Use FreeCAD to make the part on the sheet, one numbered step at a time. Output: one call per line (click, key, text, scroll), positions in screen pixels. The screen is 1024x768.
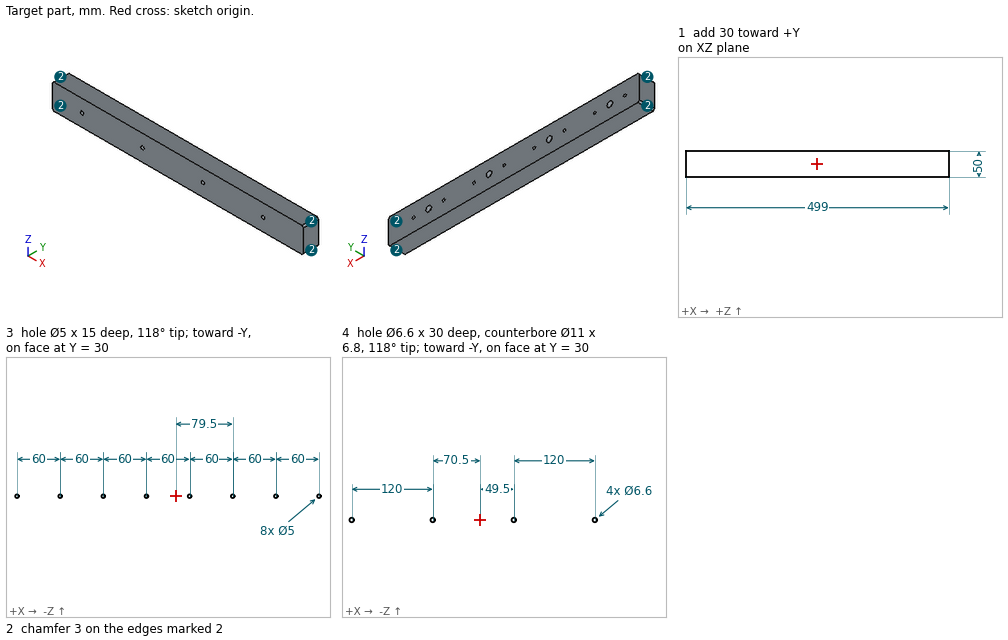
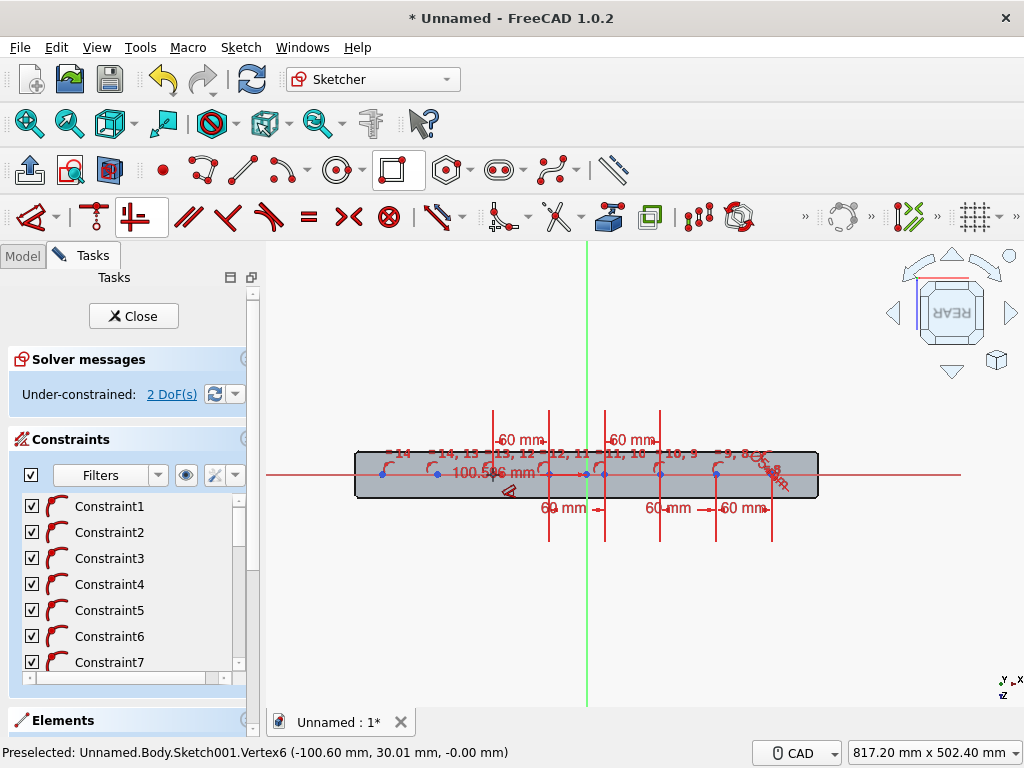
click(438, 475)
click(466, 509)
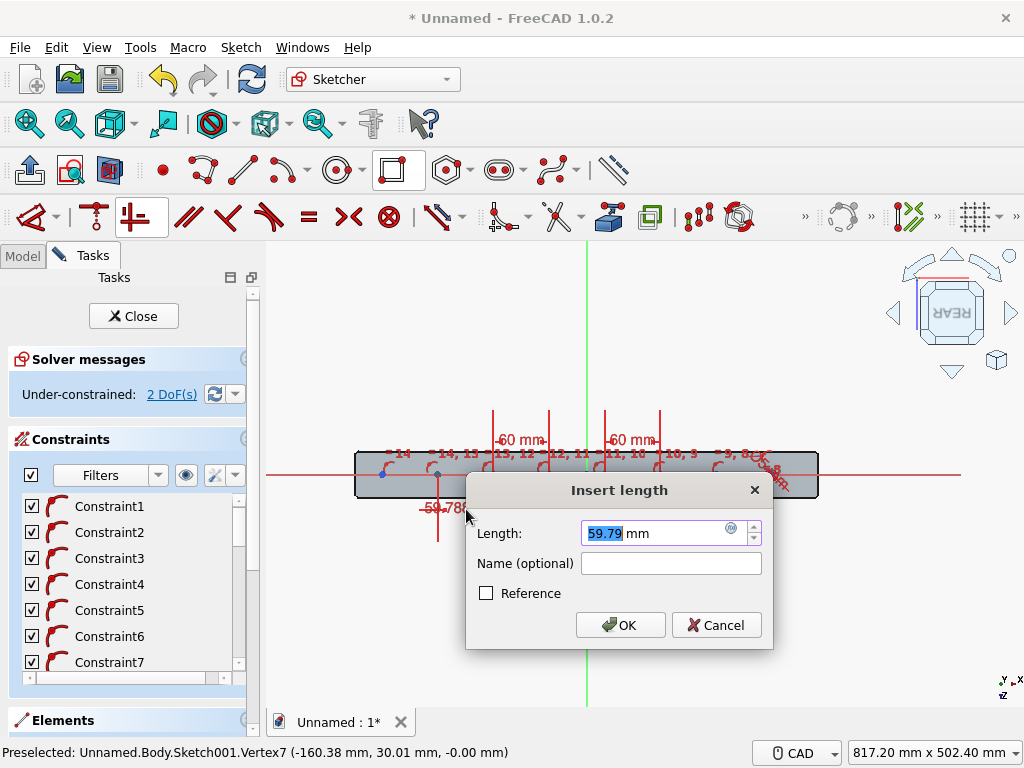
text(60)
key(Return)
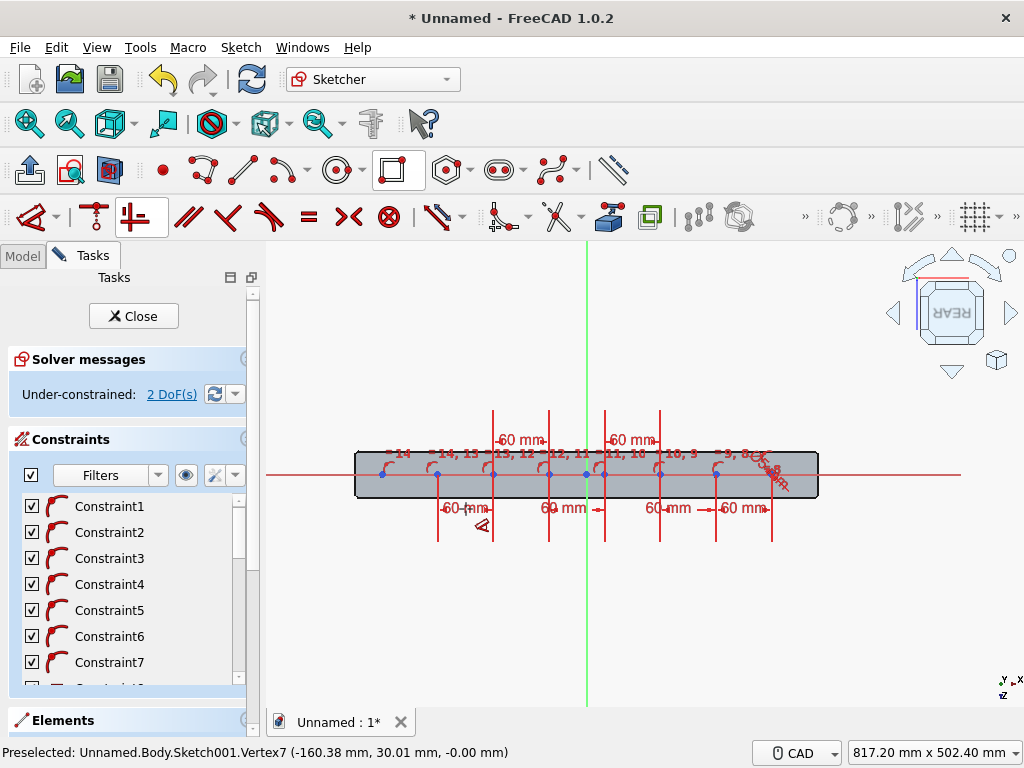
click(438, 475)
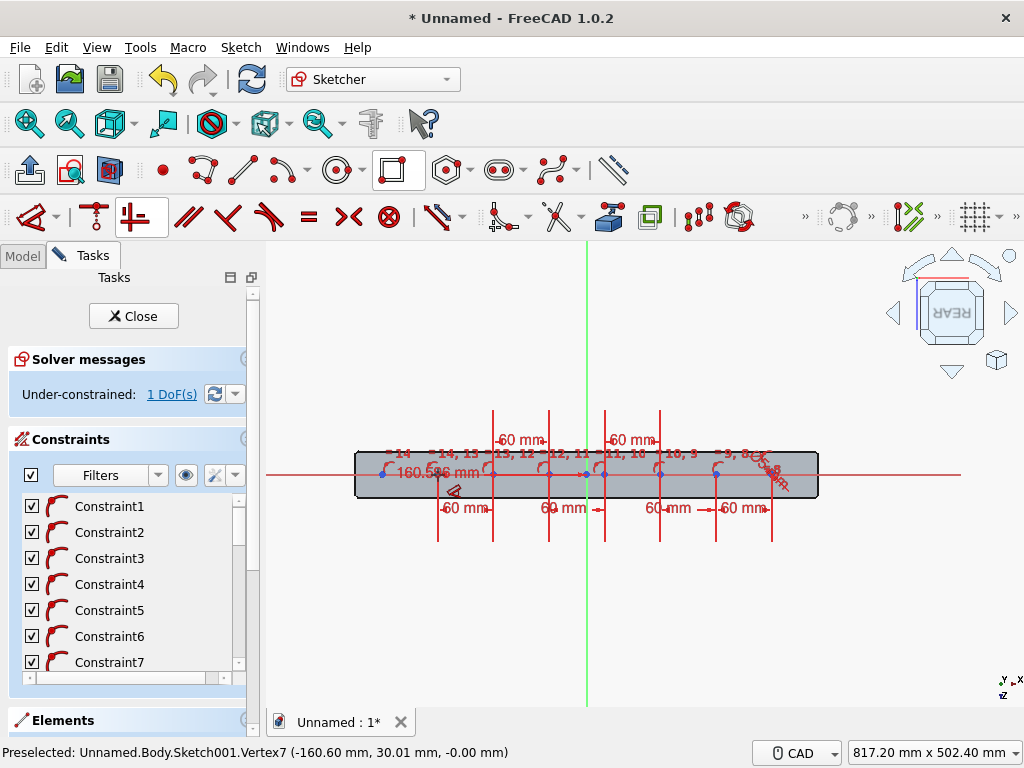
click(382, 475)
click(390, 509)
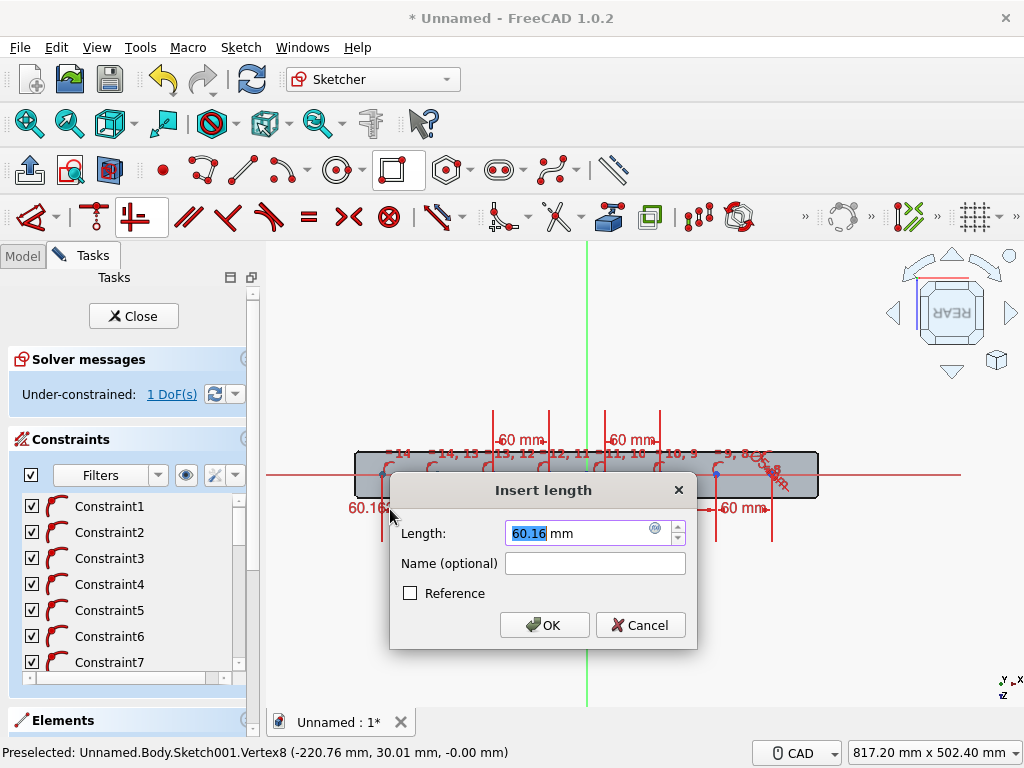
text(60)
key(Return)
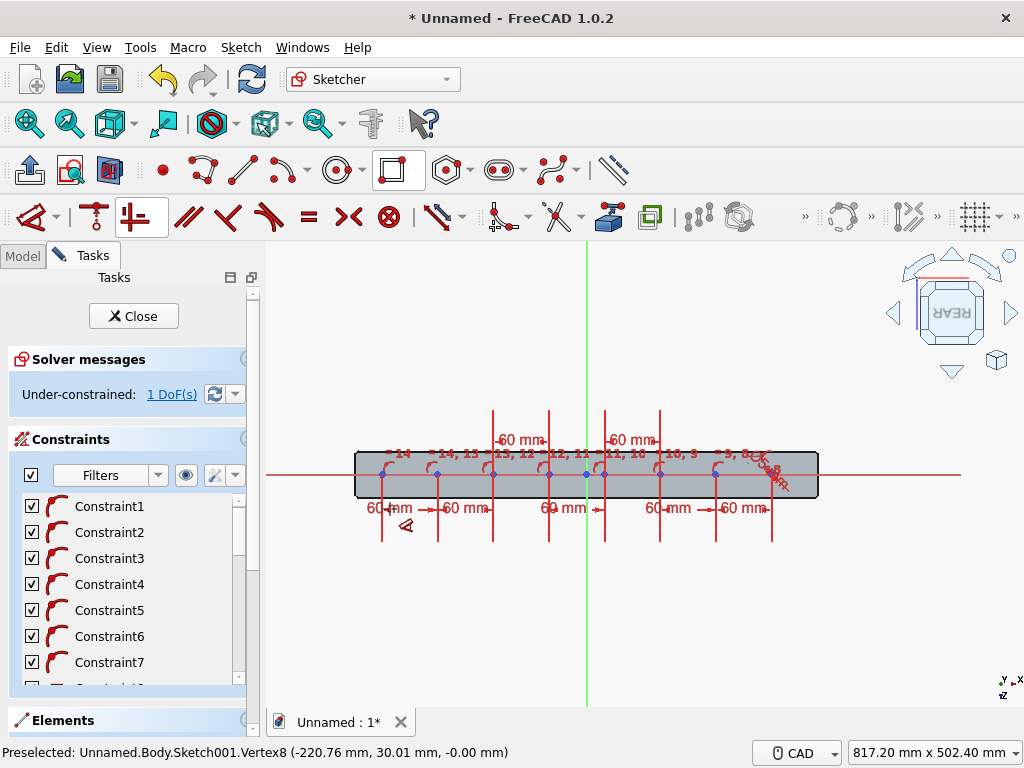
click(660, 475)
click(624, 533)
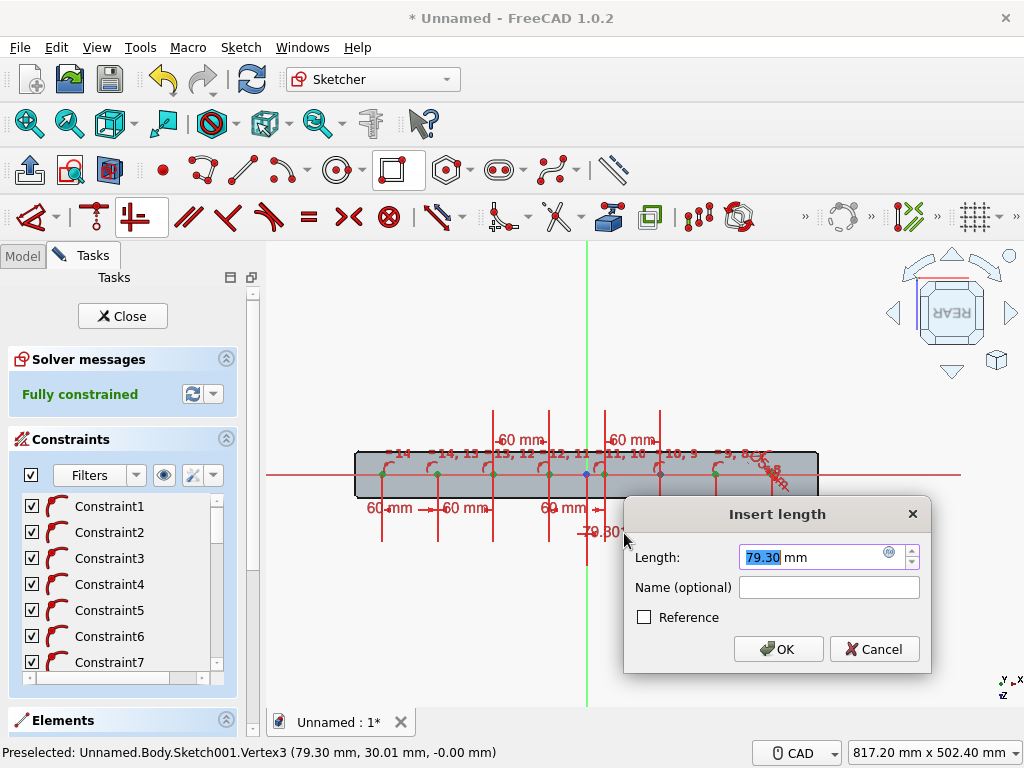
text(79.5)
key(Return)
key(Escape)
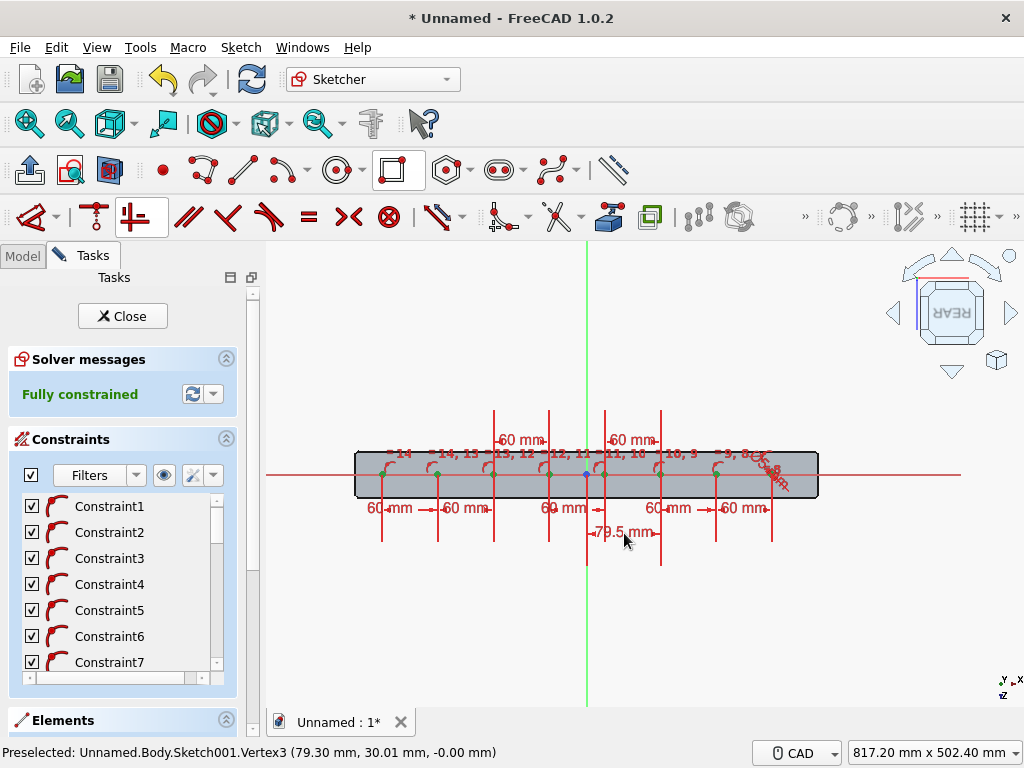
click(123, 316)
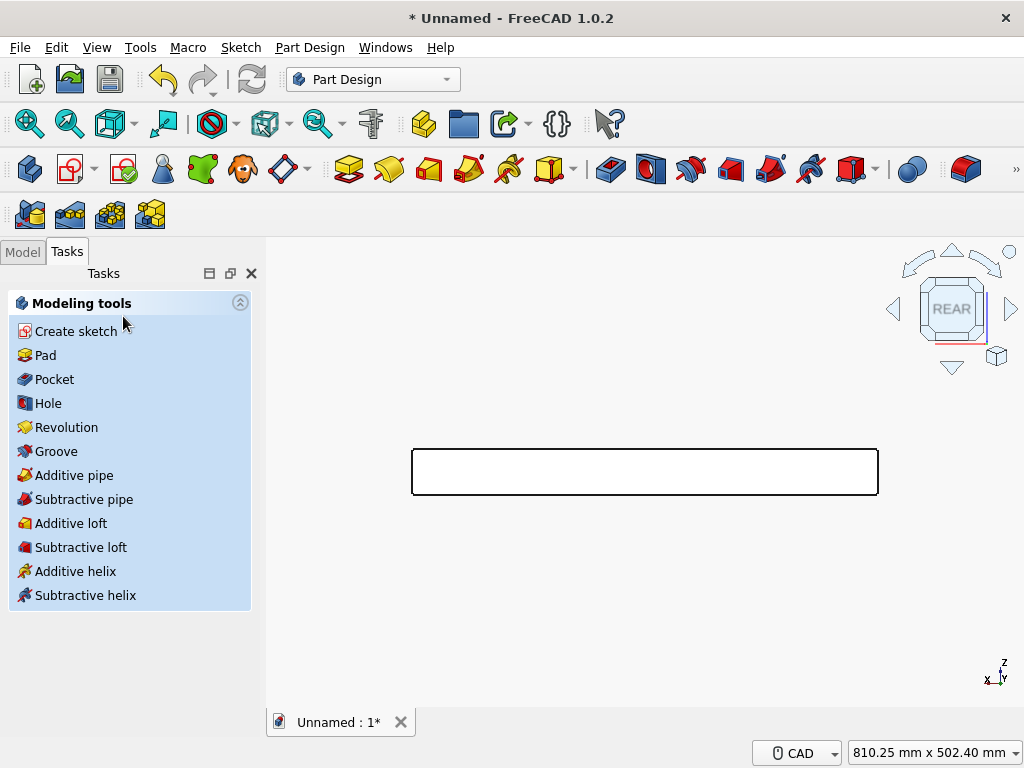
click(652, 170)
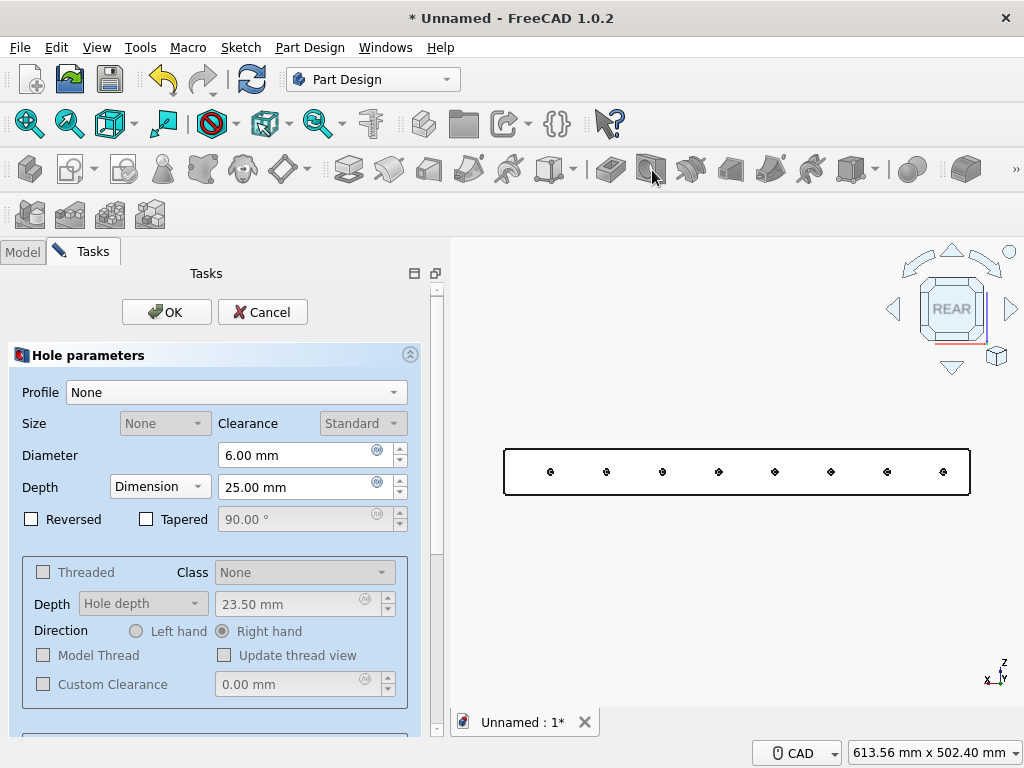
triple_click(305, 455)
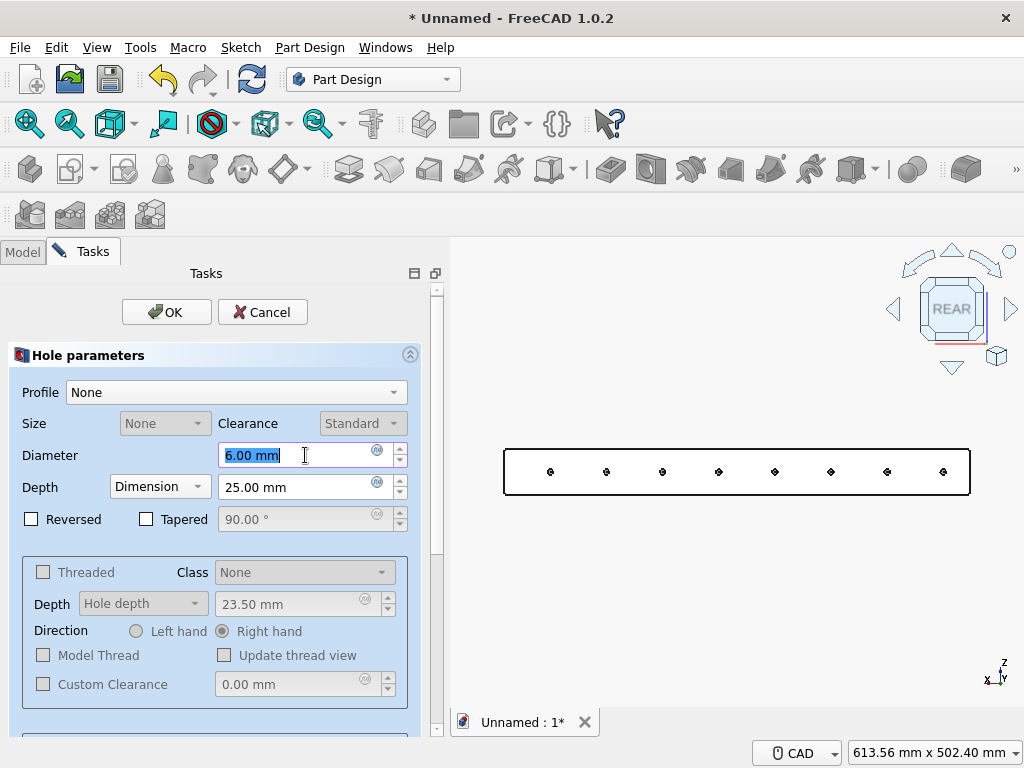
text(5)
key(Tab)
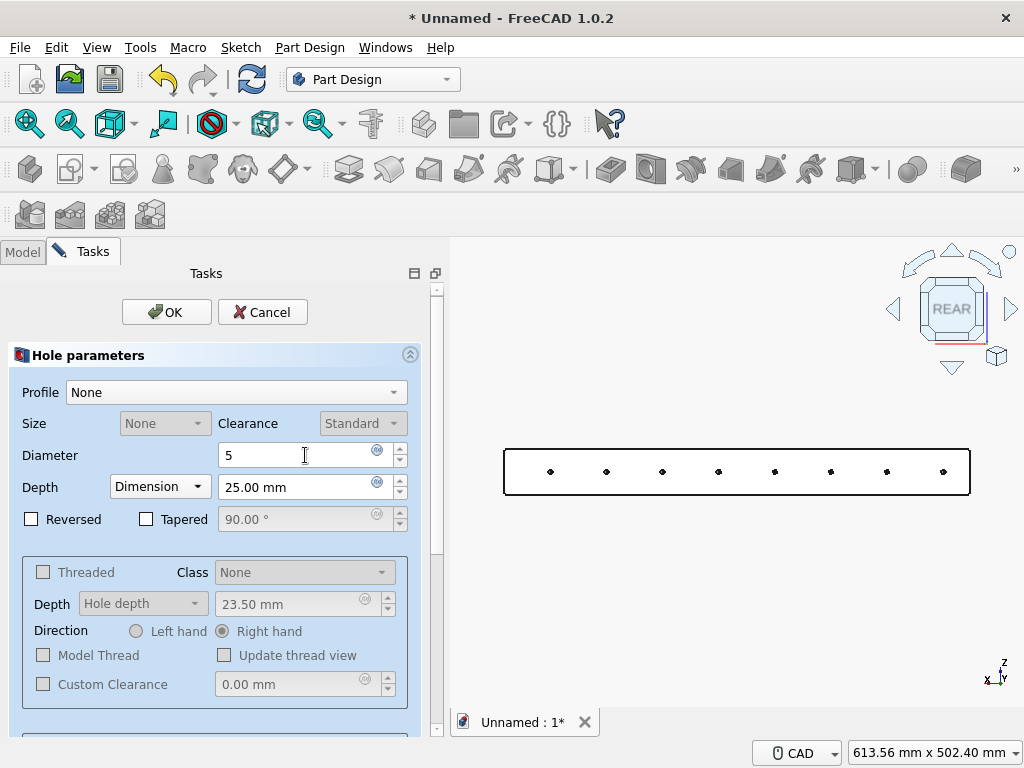
triple_click(305, 487)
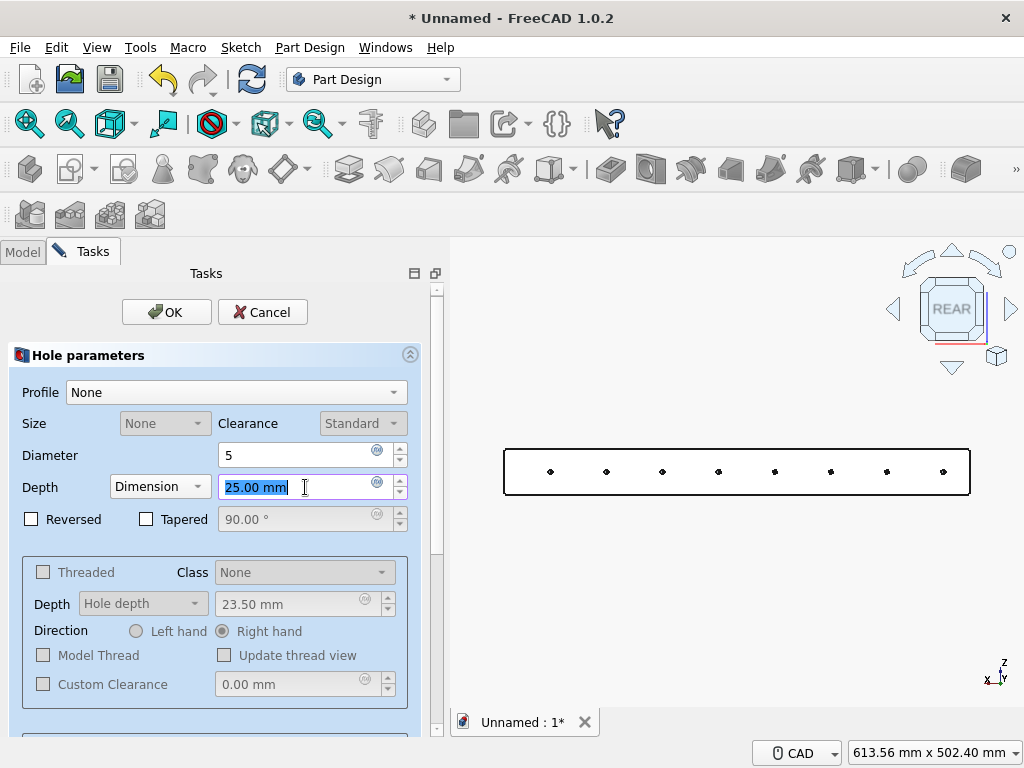
text(15)
key(Tab)